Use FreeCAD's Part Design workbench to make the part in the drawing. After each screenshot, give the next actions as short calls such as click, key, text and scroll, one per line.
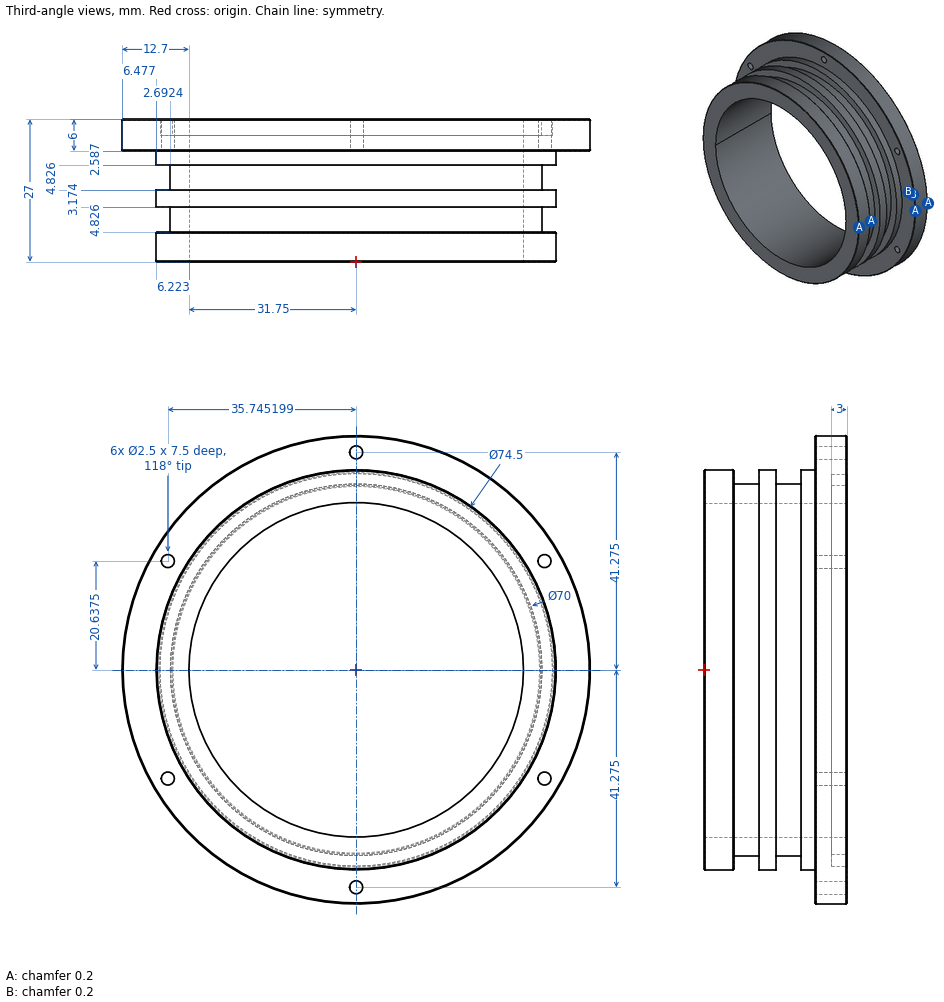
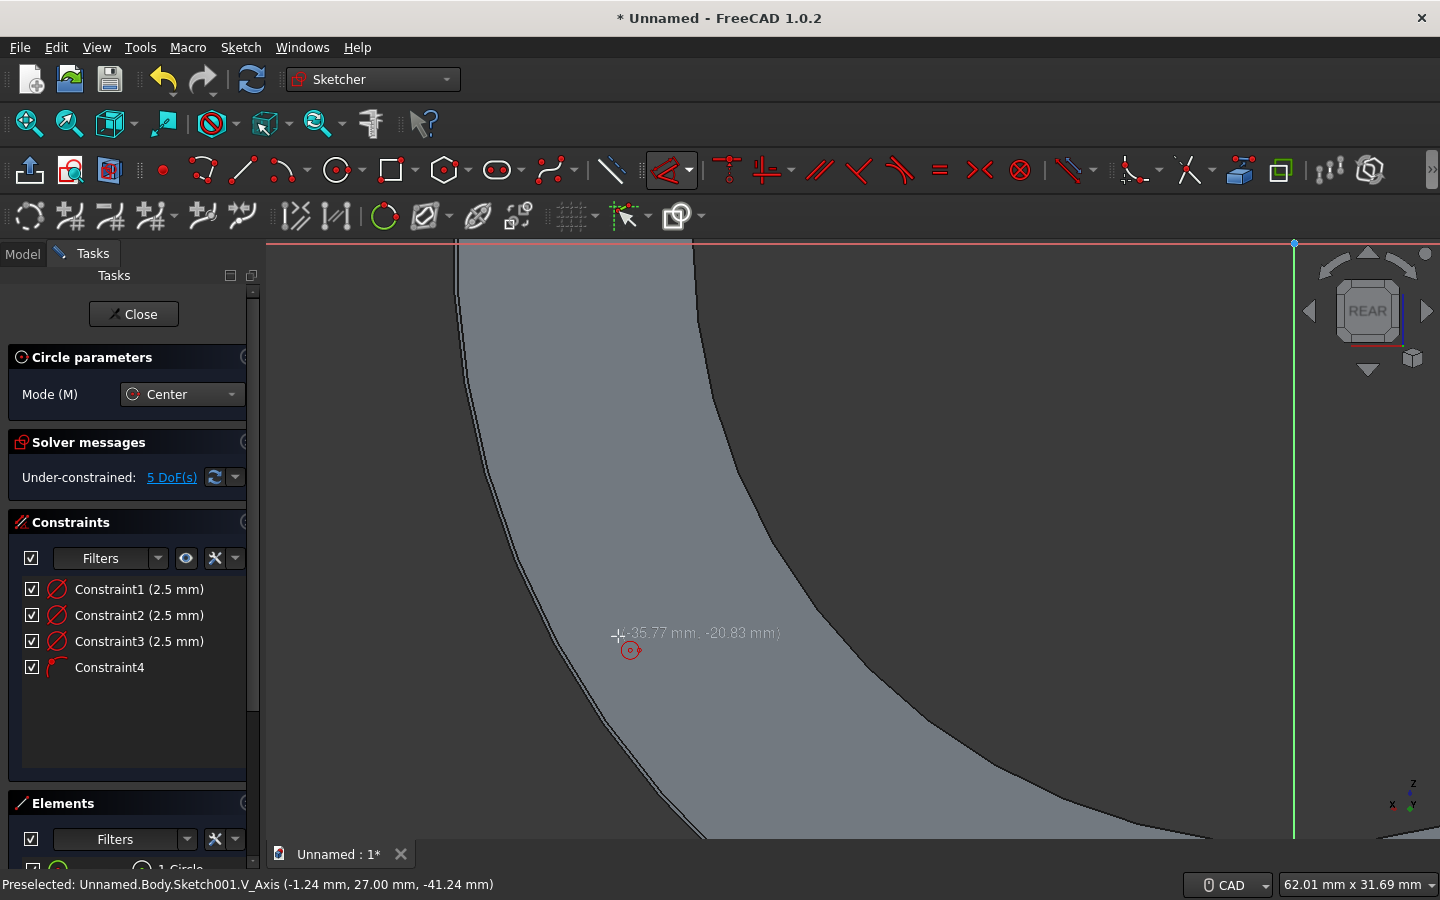
scroll(618, 636, down, 7)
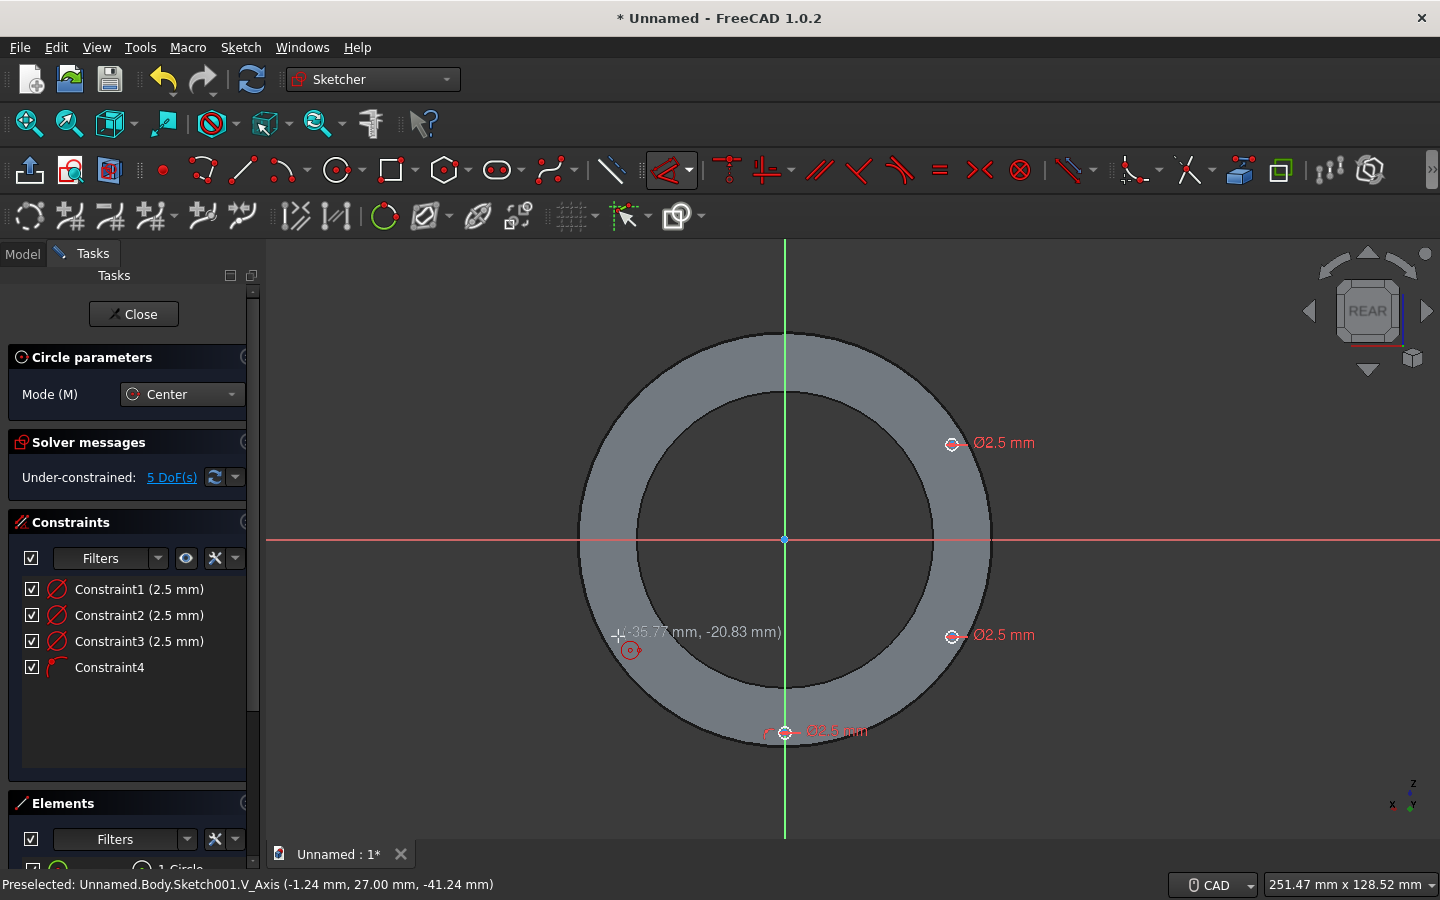
click(618, 636)
move(622, 632)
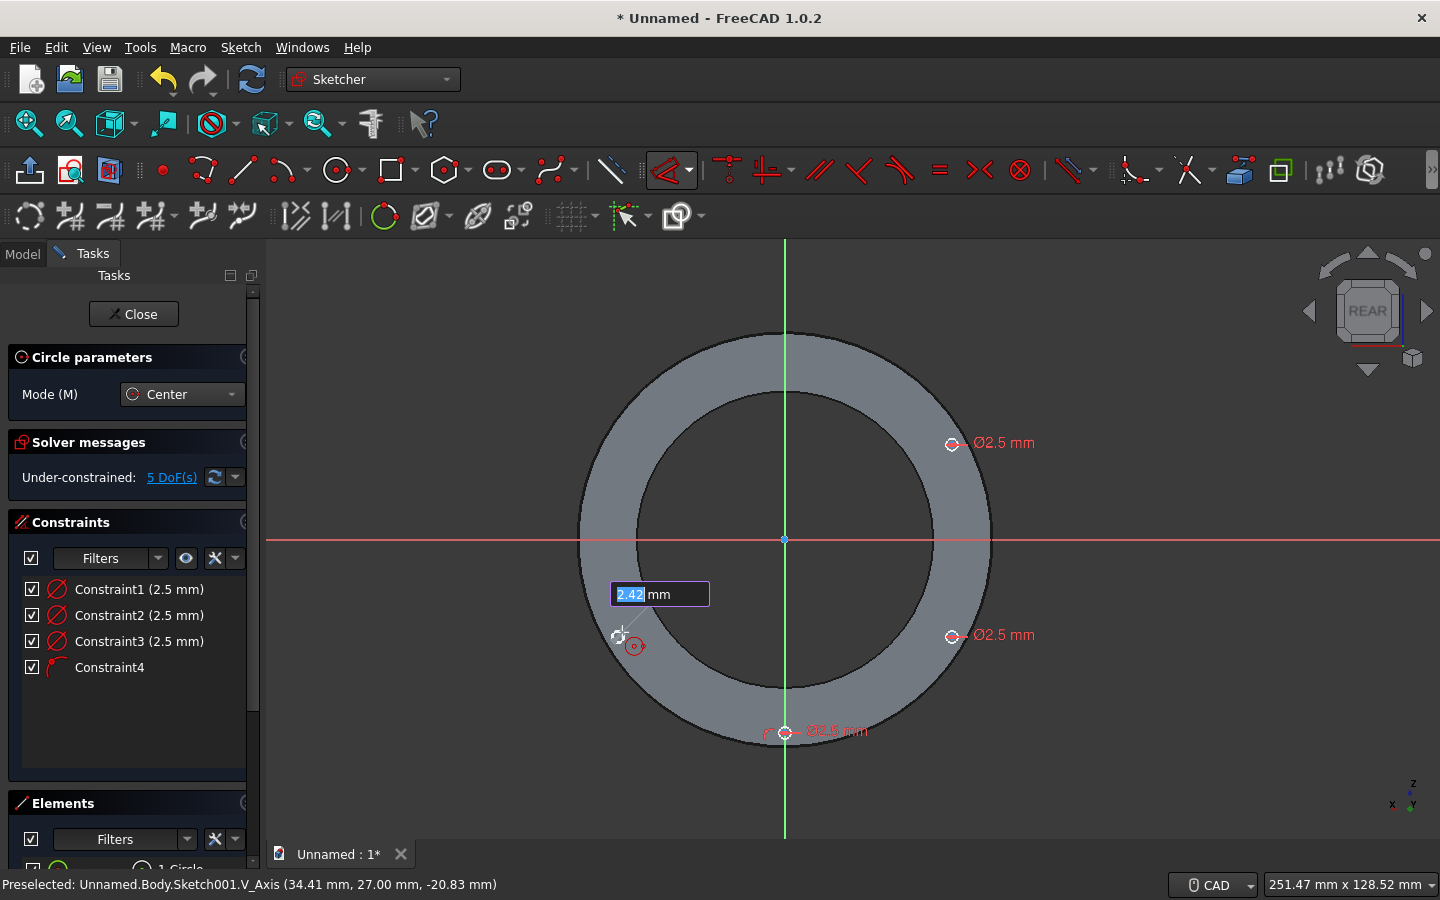
text(2.5)
key(Return)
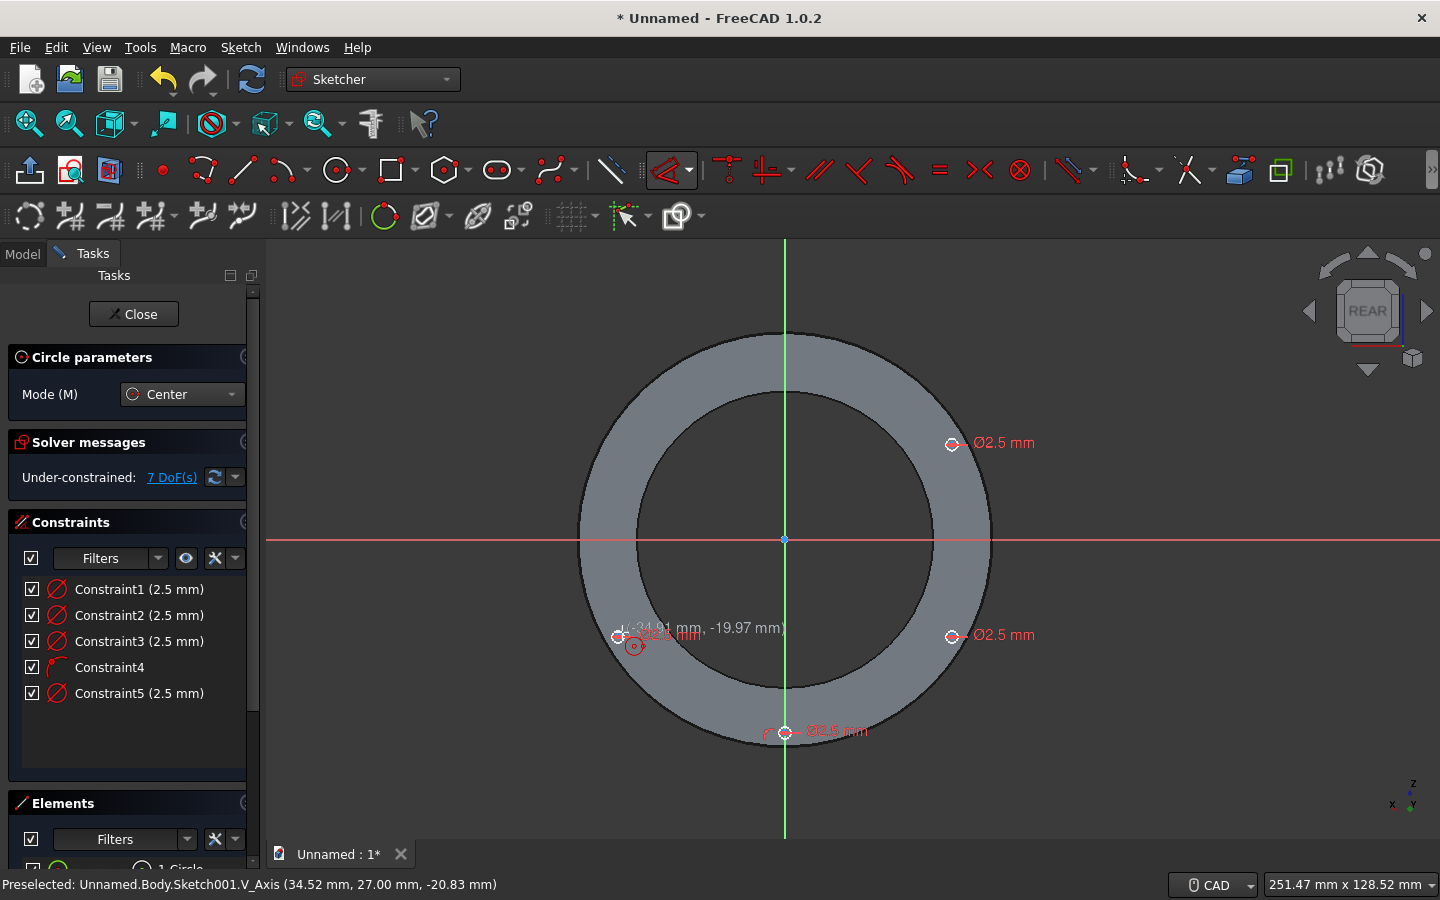
scroll(618, 443, up, 7)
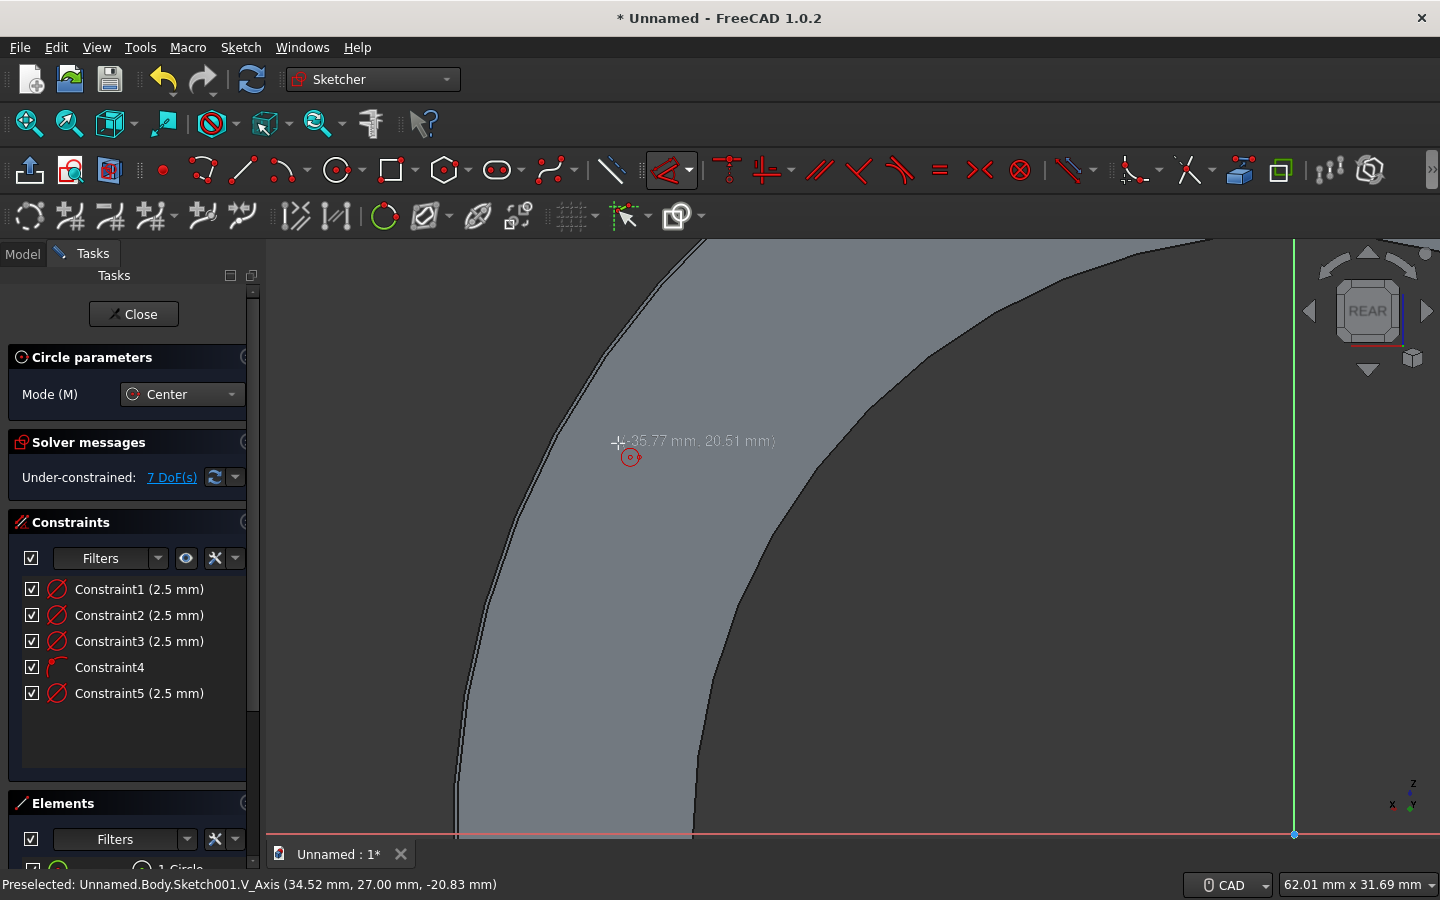
scroll(618, 442, down, 7)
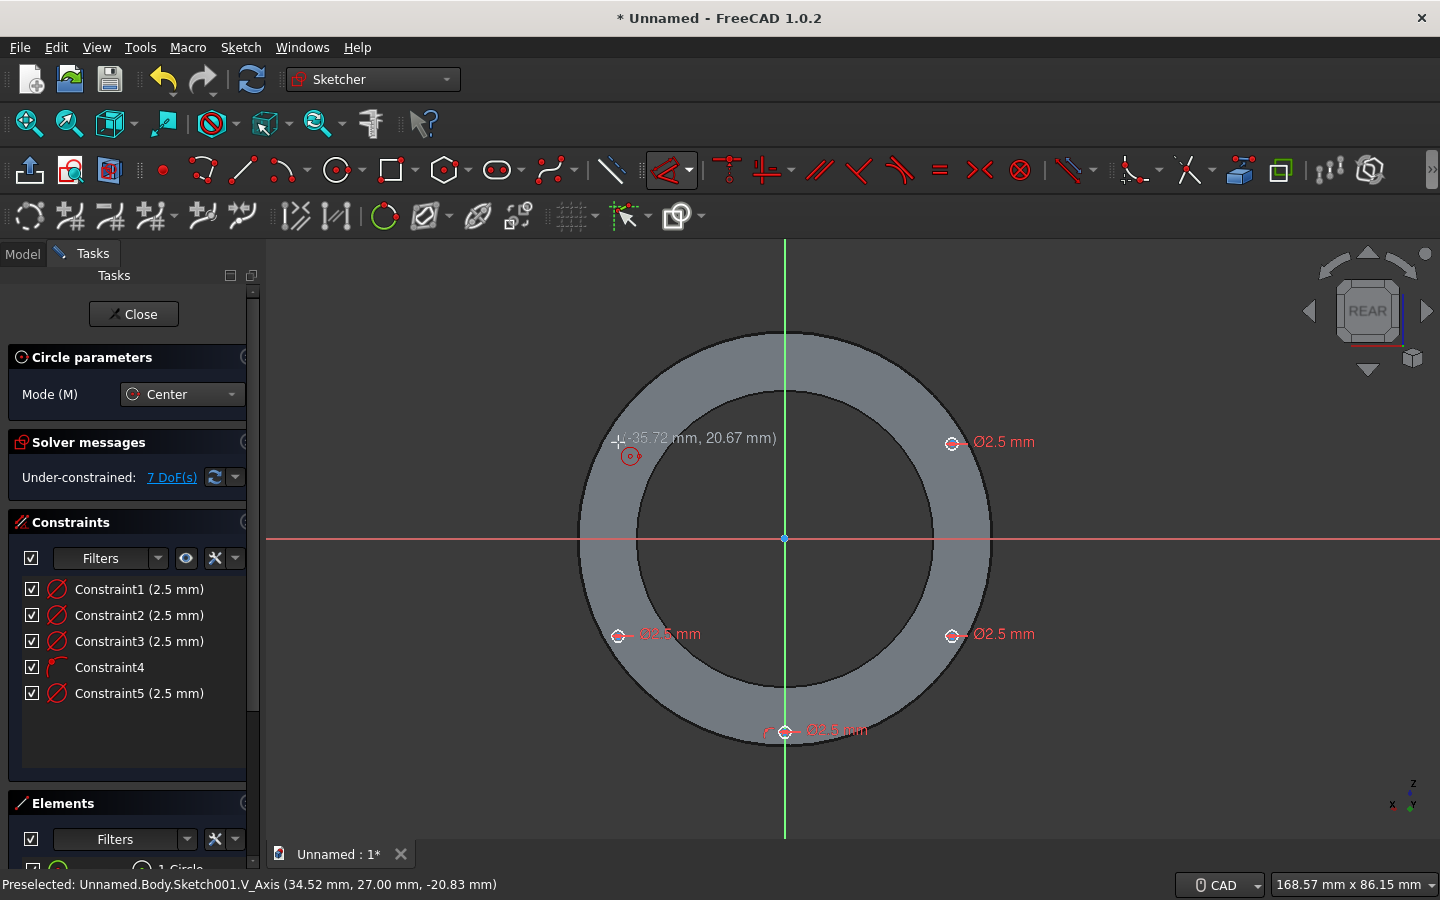
click(618, 443)
move(622, 439)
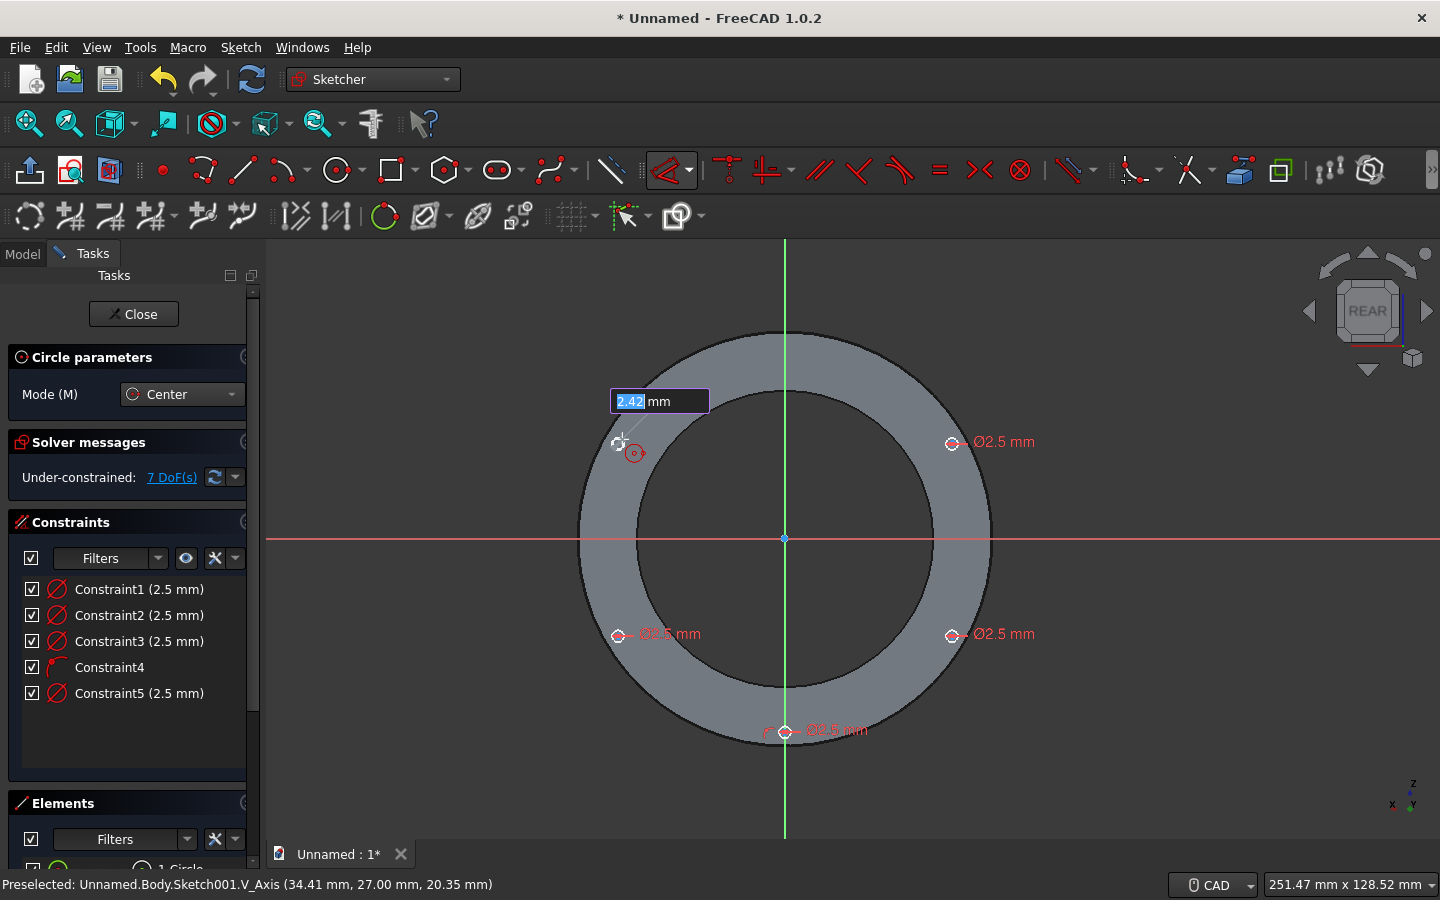
text(2.5)
key(Return)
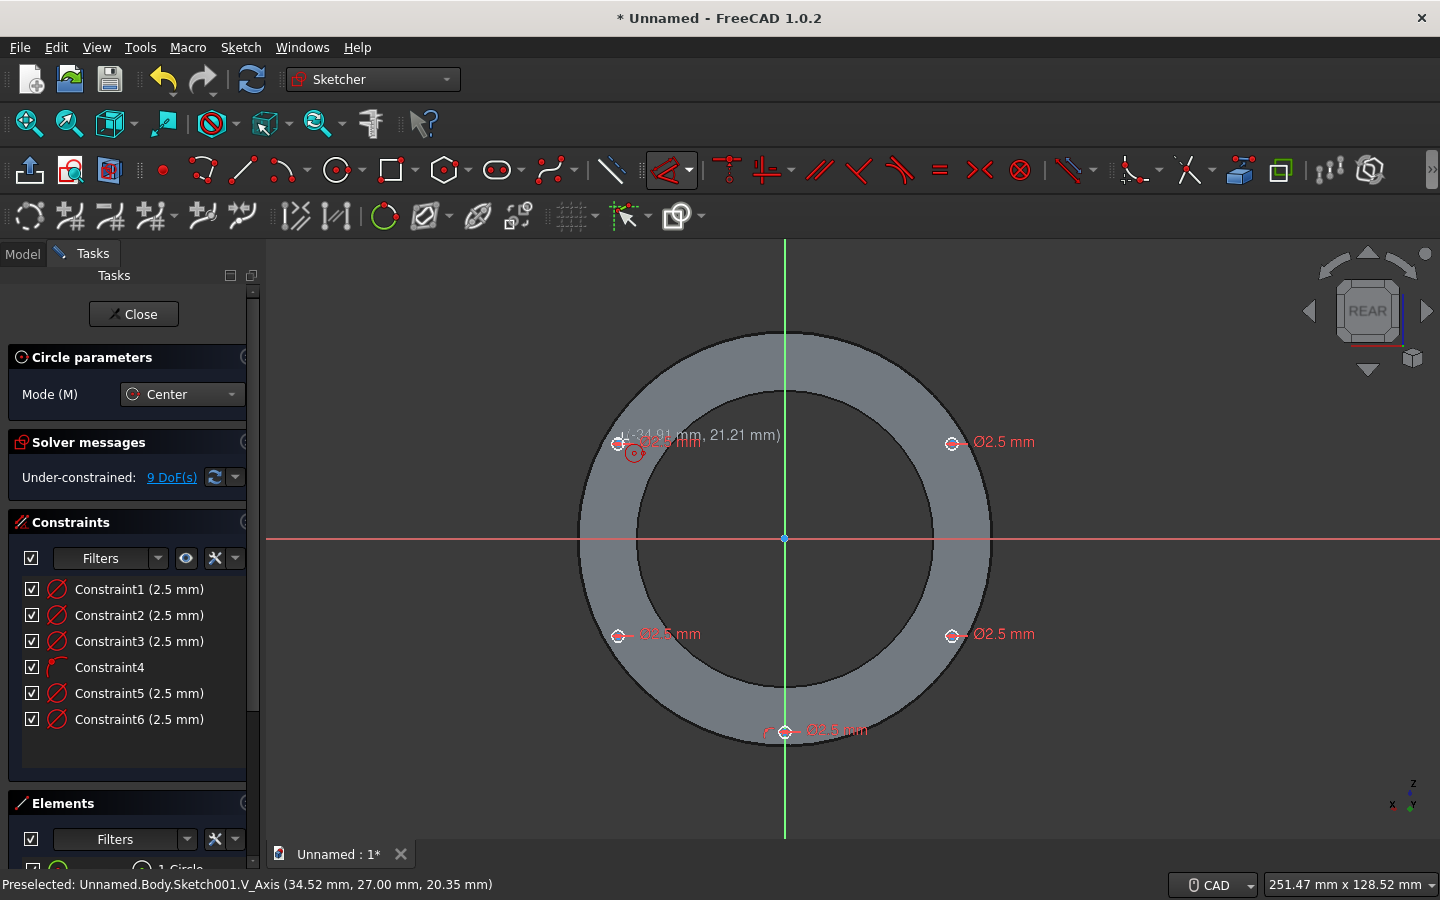
scroll(785, 346, up, 7)